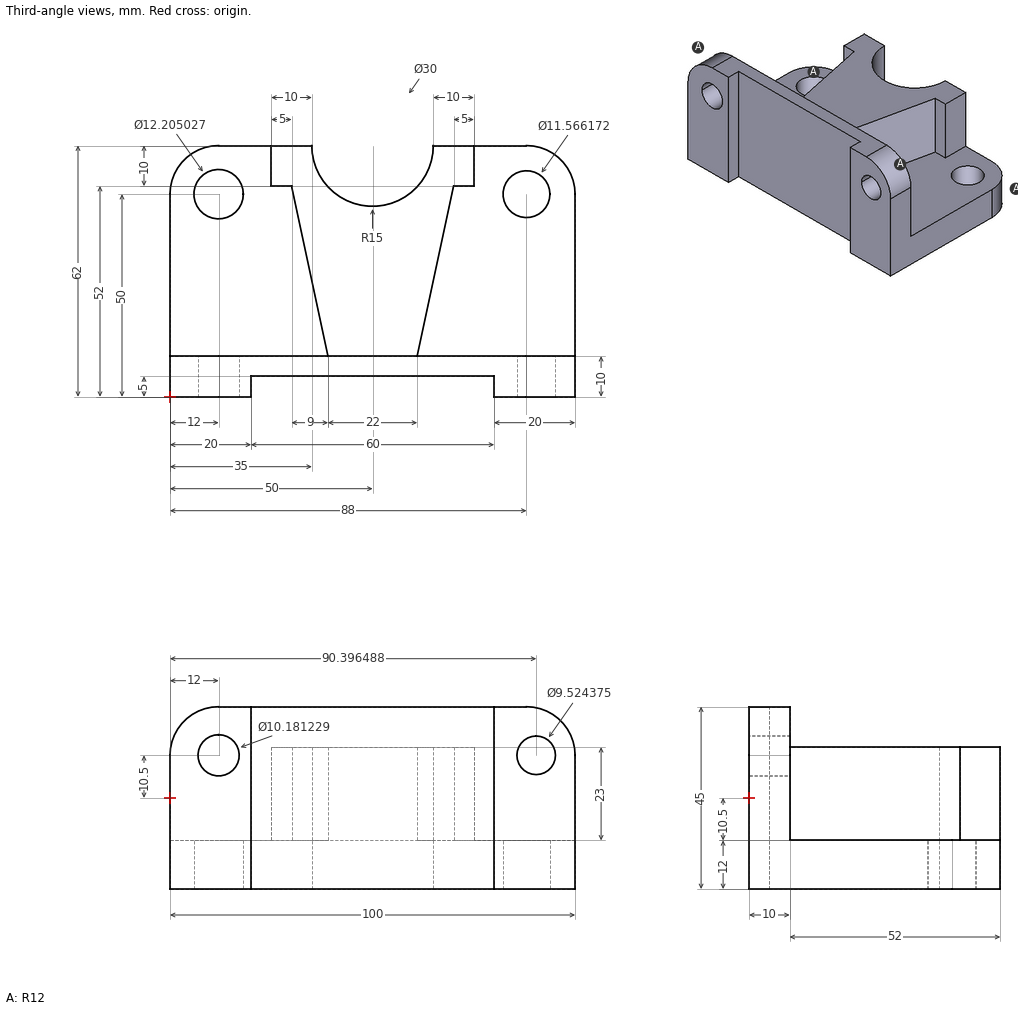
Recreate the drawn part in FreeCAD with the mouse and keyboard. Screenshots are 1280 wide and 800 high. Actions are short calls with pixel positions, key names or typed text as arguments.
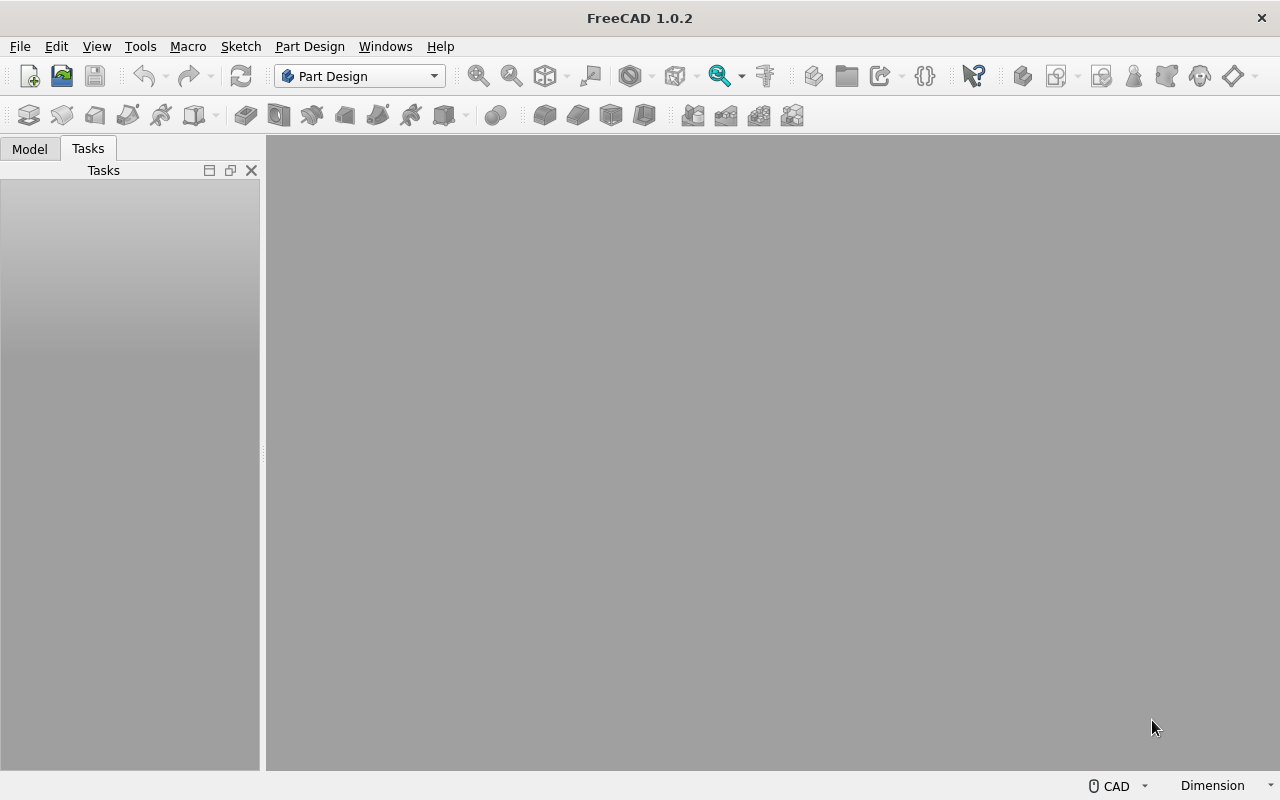
key(ctrl+n)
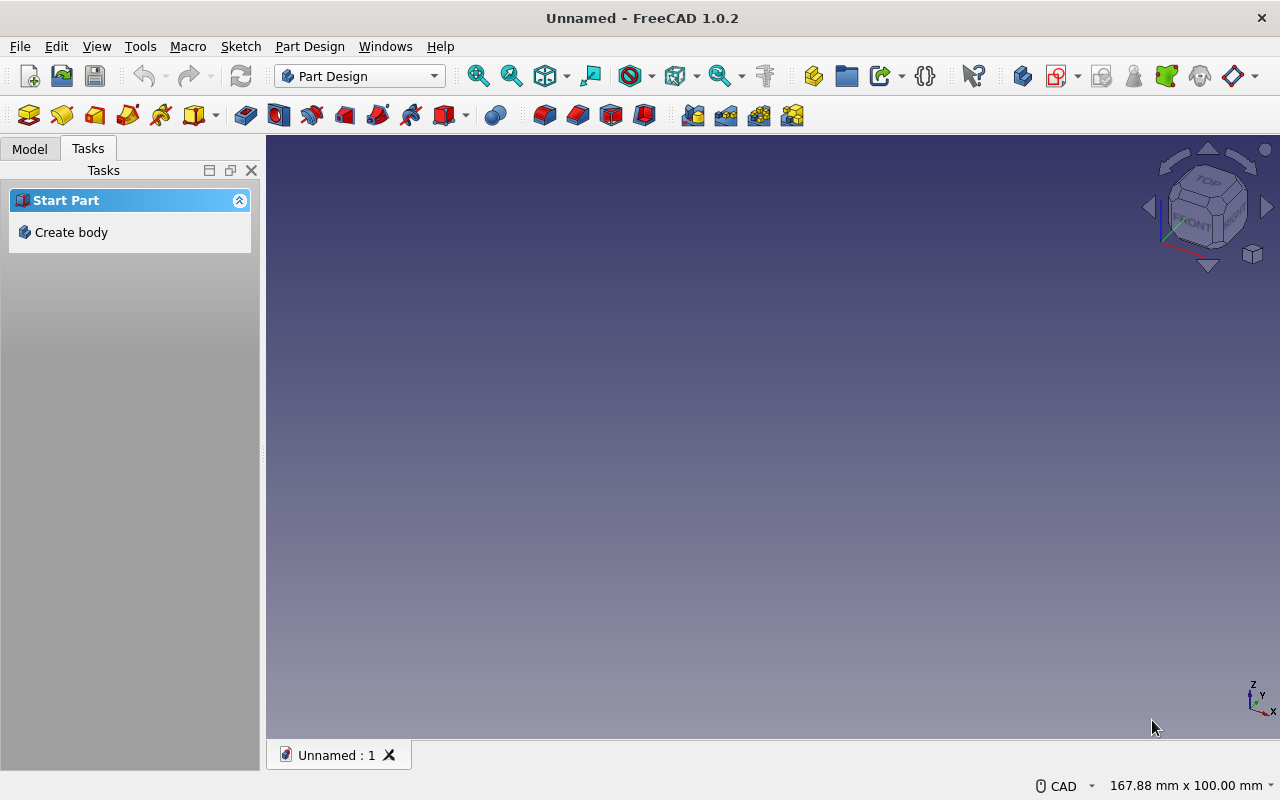
click(1056, 76)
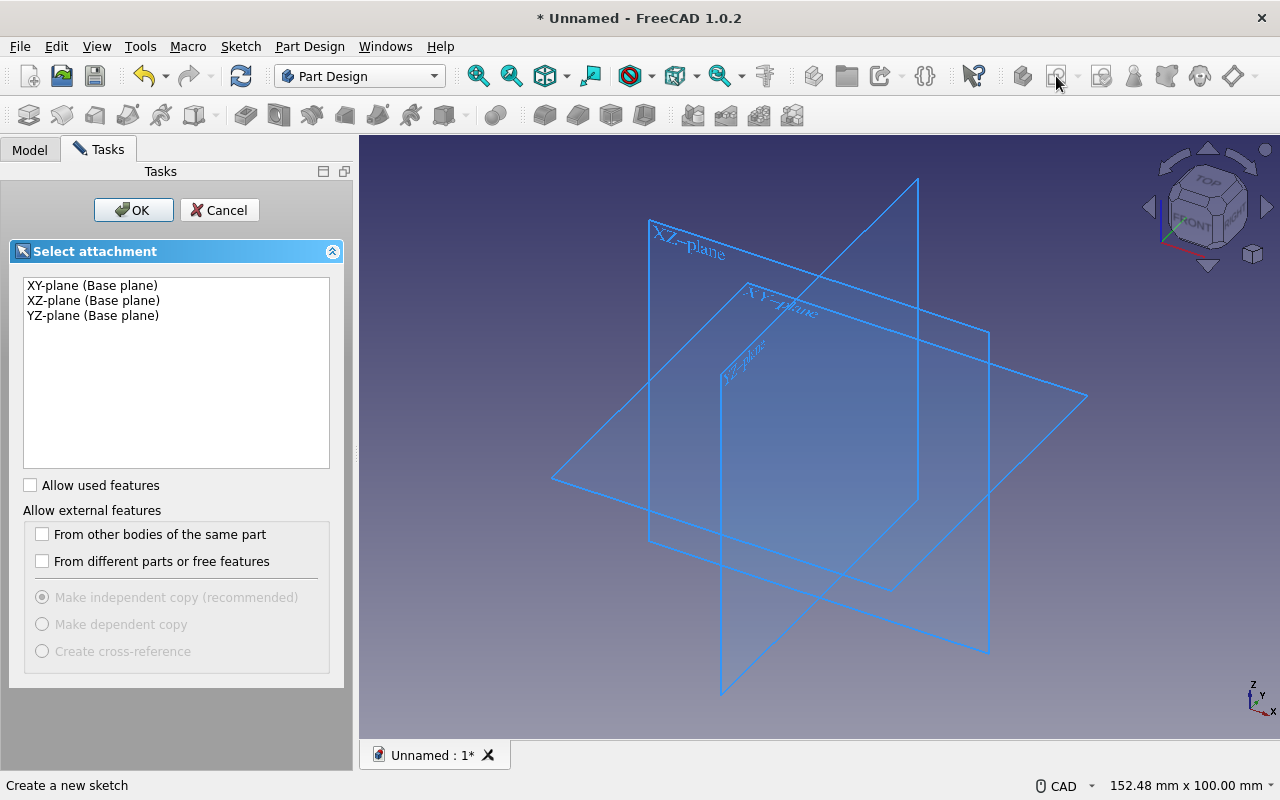
click(84, 286)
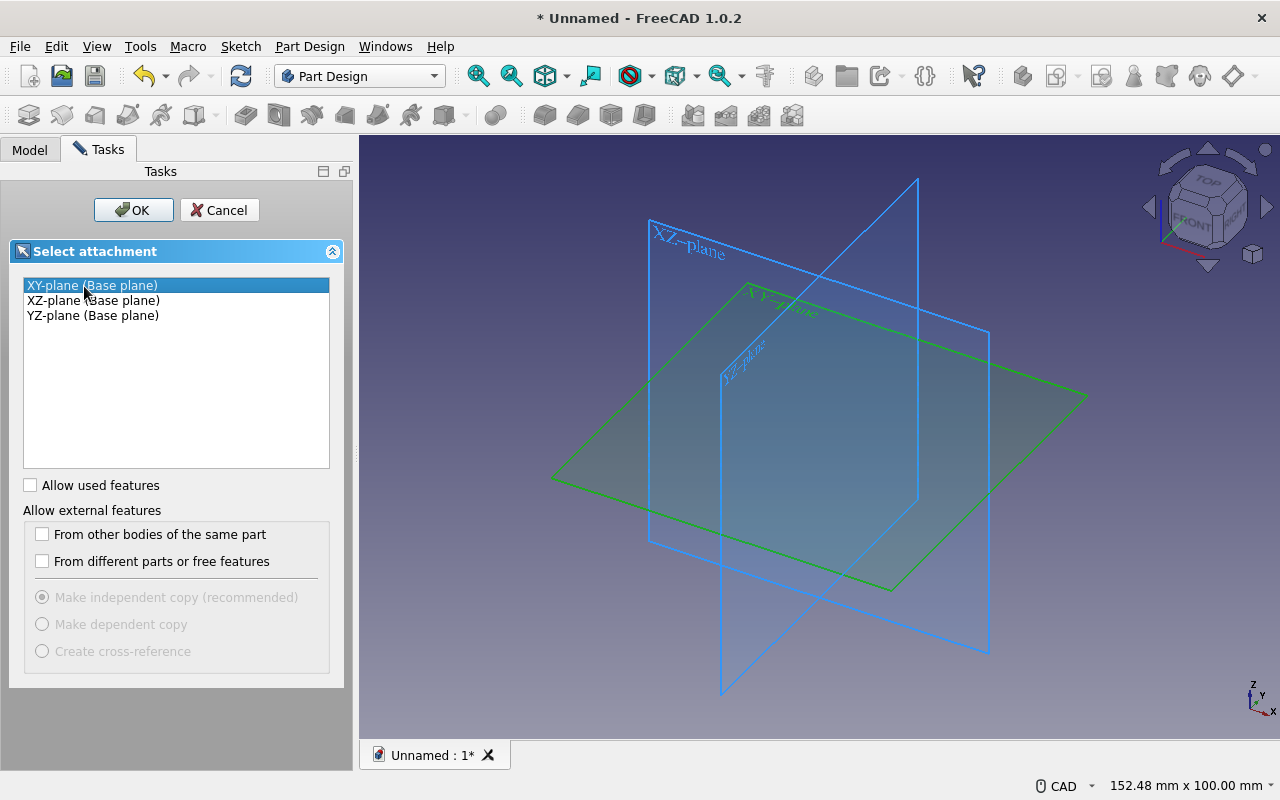
click(134, 210)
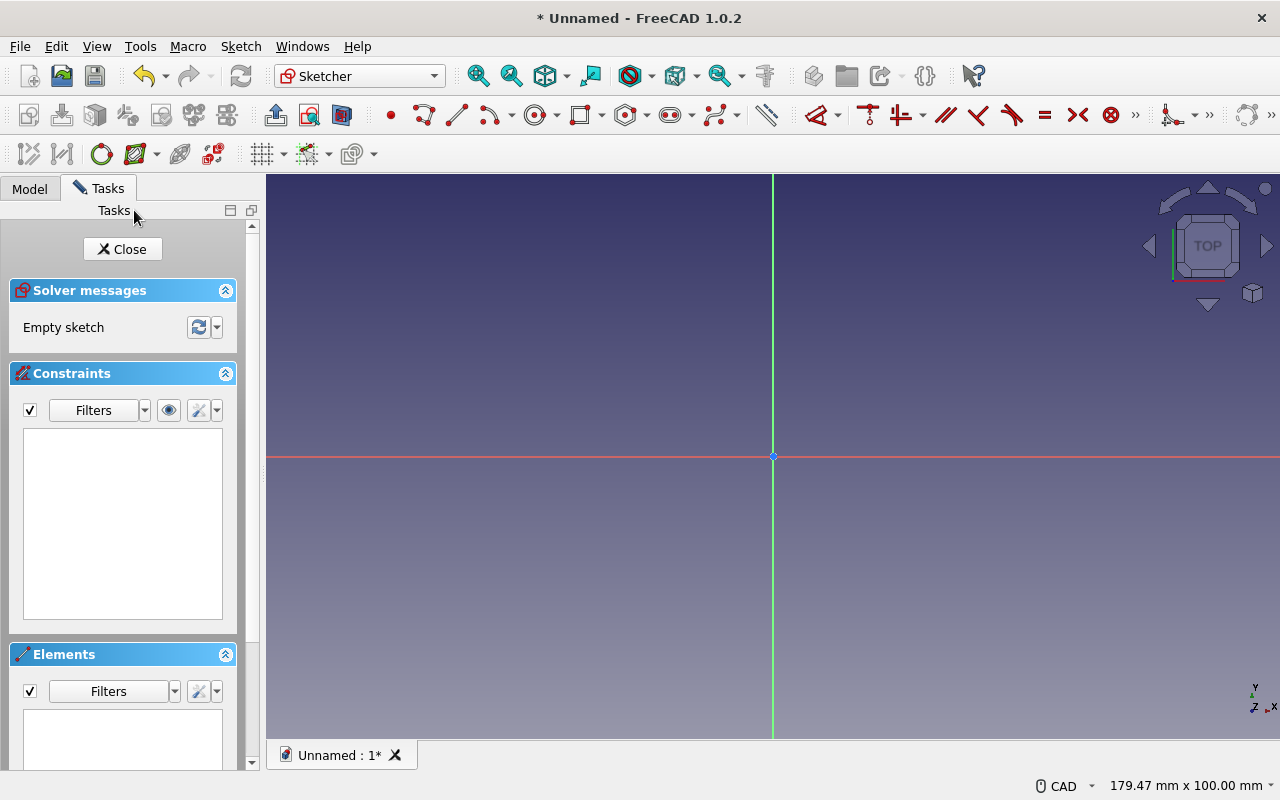
scroll(294, 514, down, 2)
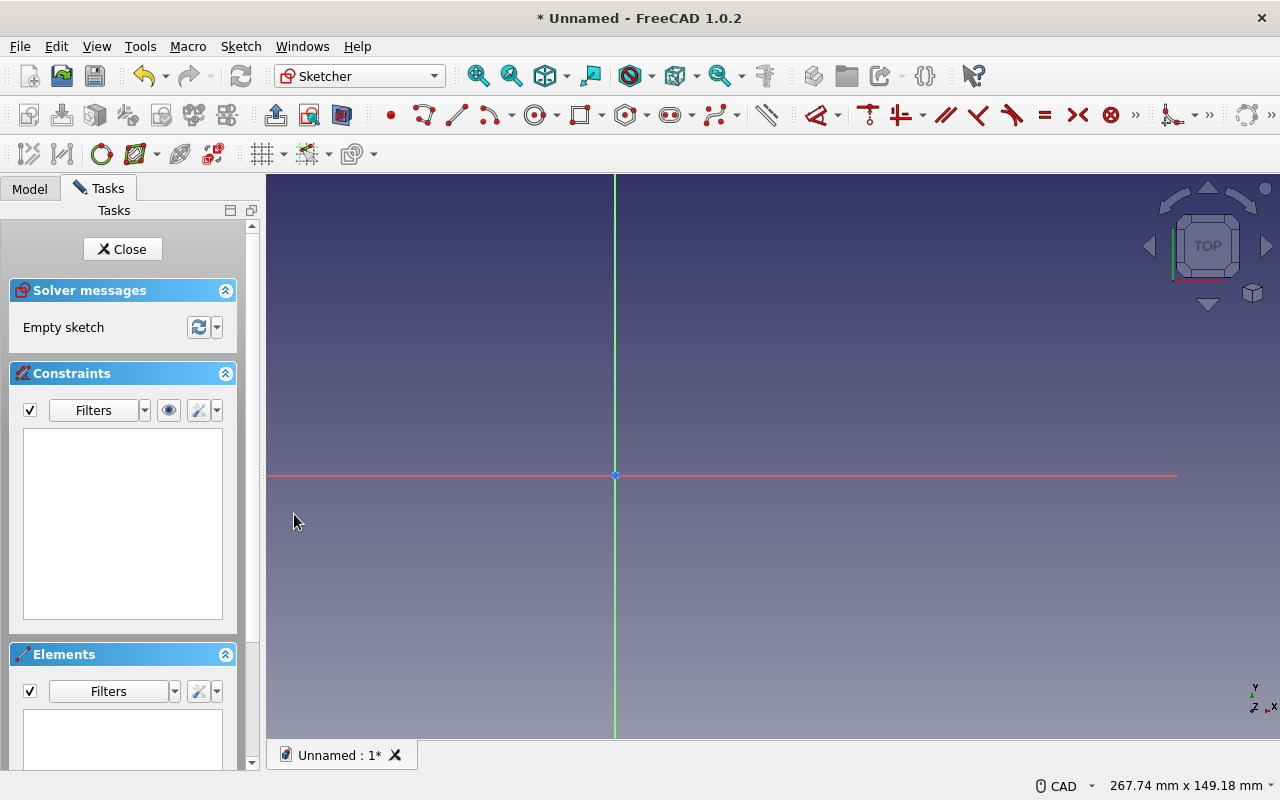
scroll(1008, 457, up, 2)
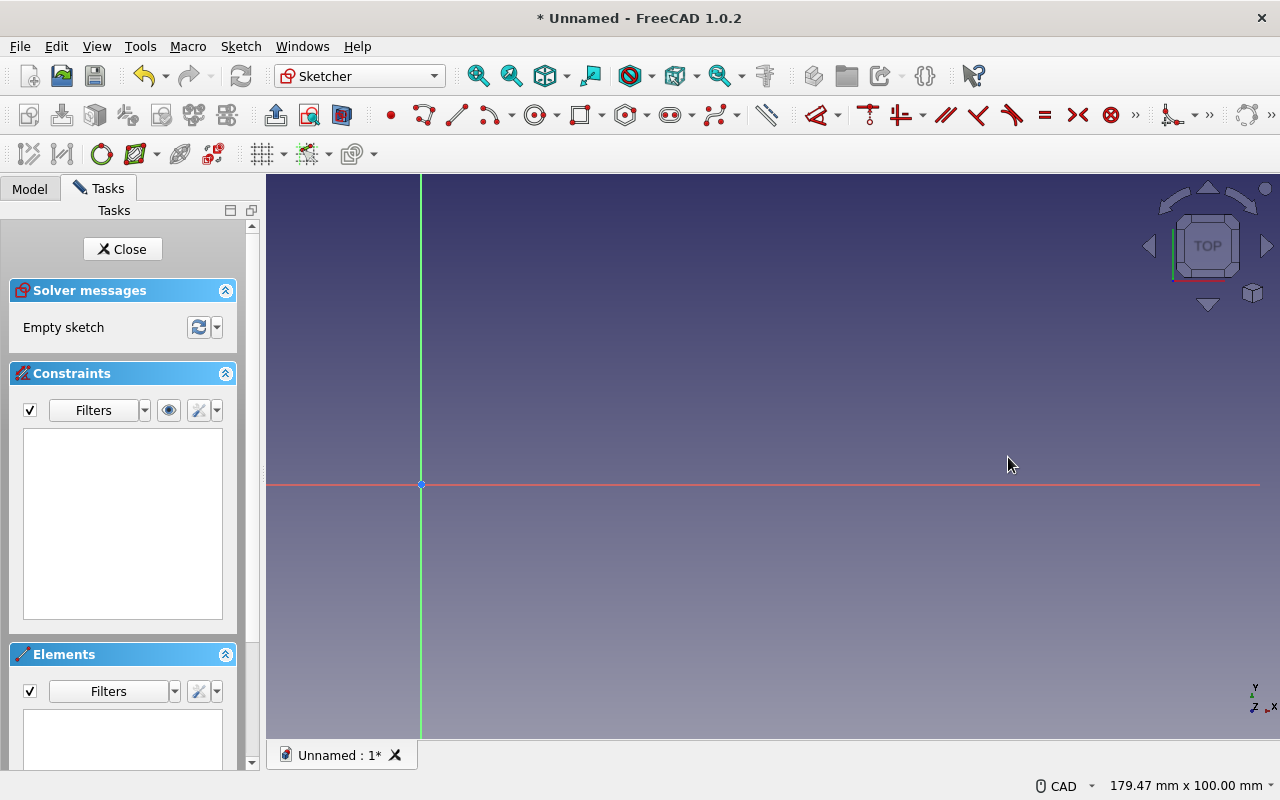
key(g)
key(m)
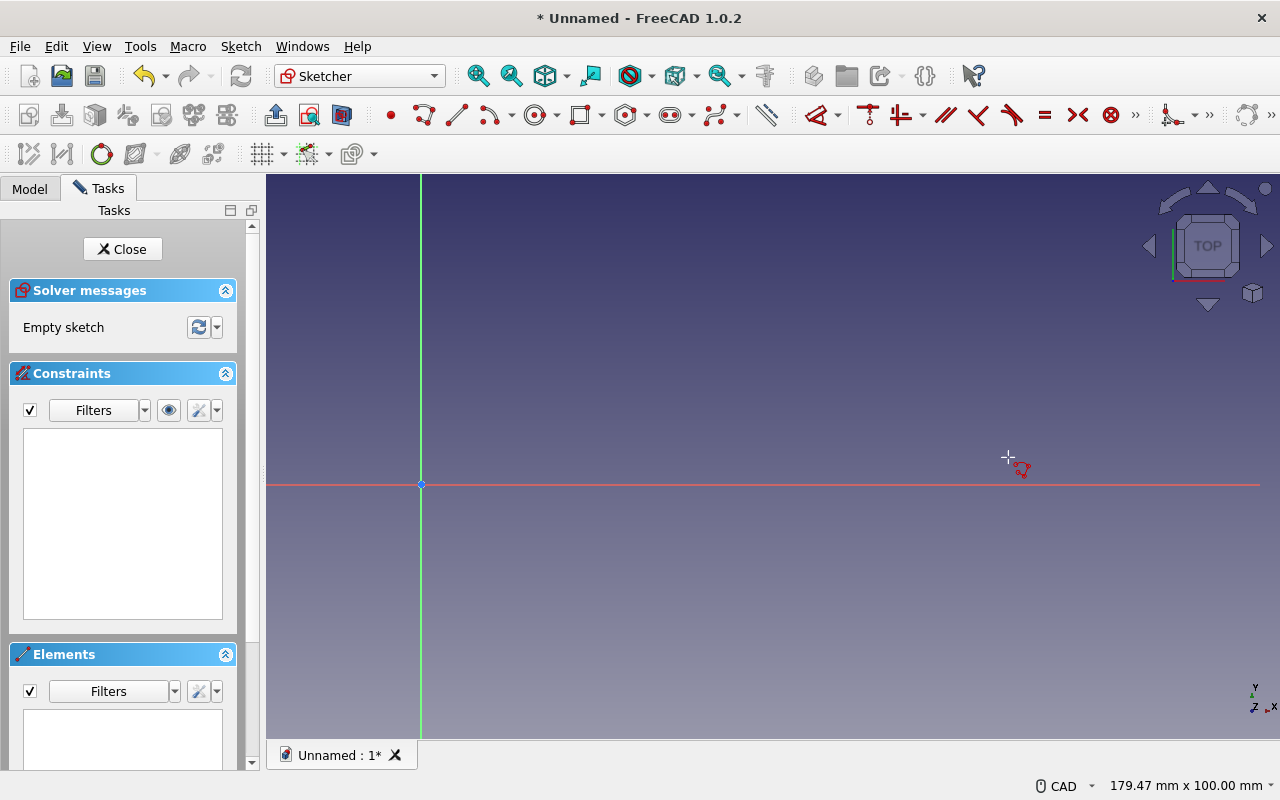
click(421, 485)
click(534, 476)
click(534, 456)
click(873, 456)
click(873, 485)
click(986, 476)
click(986, 428)
click(430, 428)
click(421, 485)
key(Escape)
key(Escape)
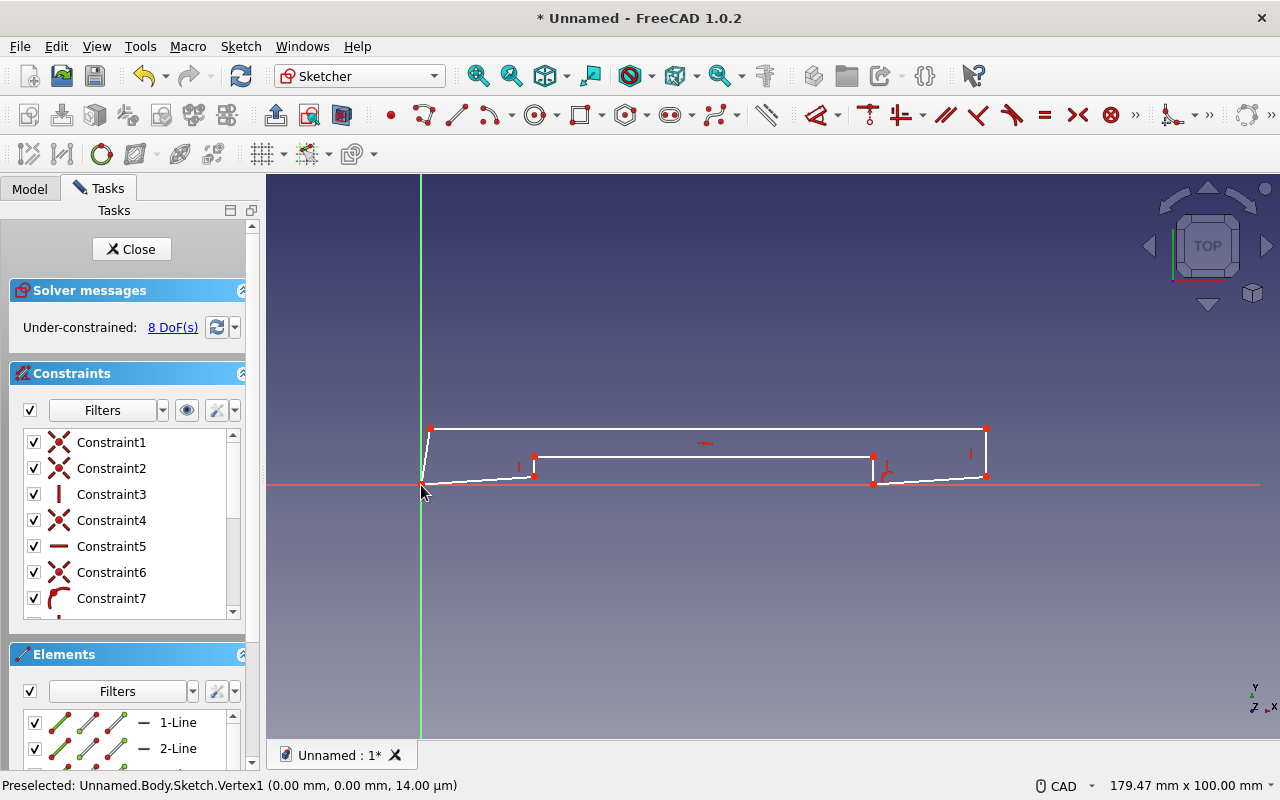
click(455, 482)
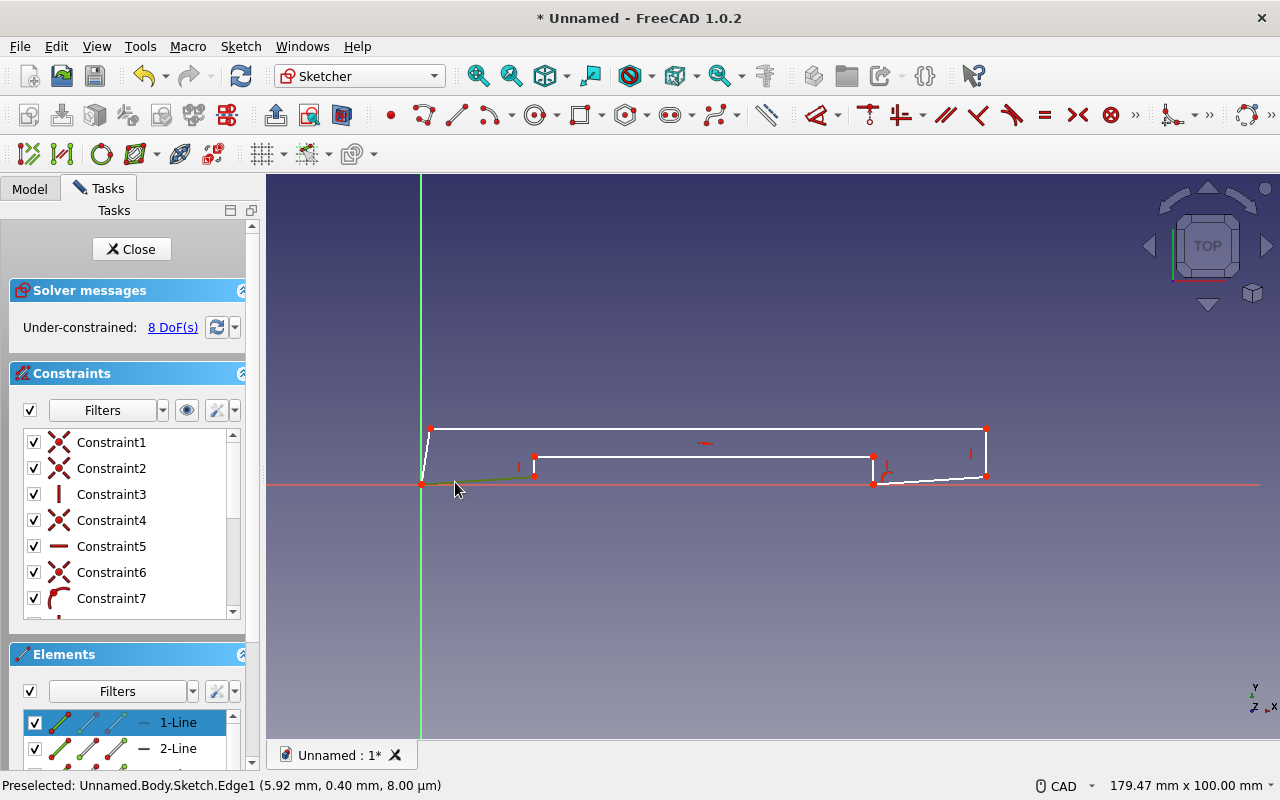
key(h)